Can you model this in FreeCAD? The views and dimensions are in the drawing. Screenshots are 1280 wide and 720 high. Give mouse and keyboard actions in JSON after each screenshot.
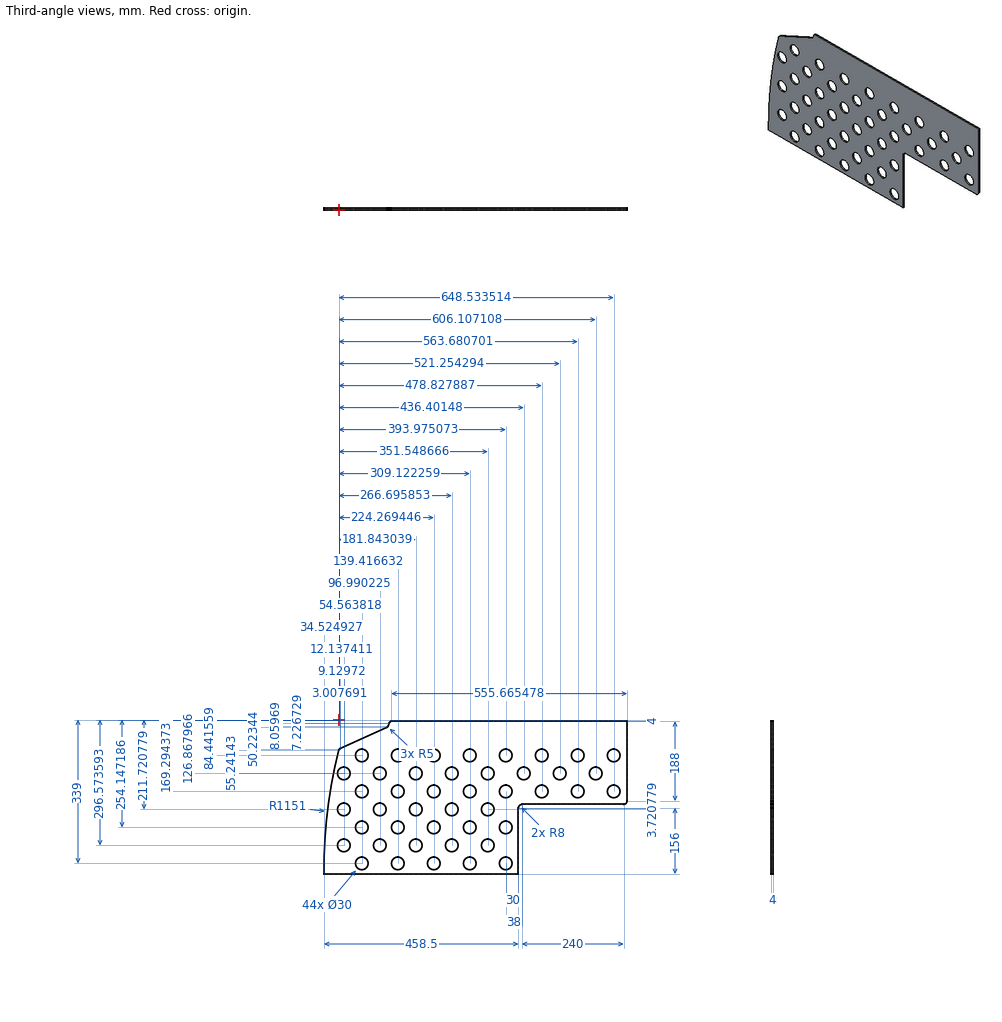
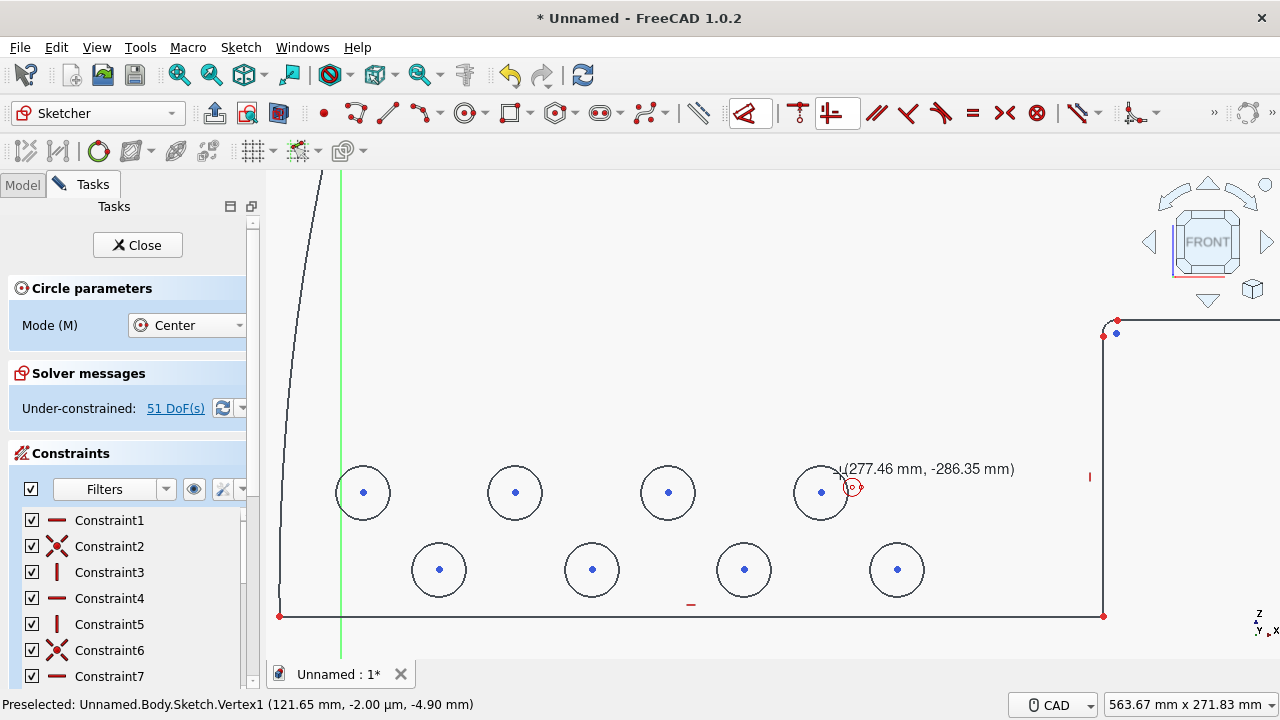
{"action": "left_click", "coordinate": [439, 416]}
{"action": "left_click", "coordinate": [458, 397]}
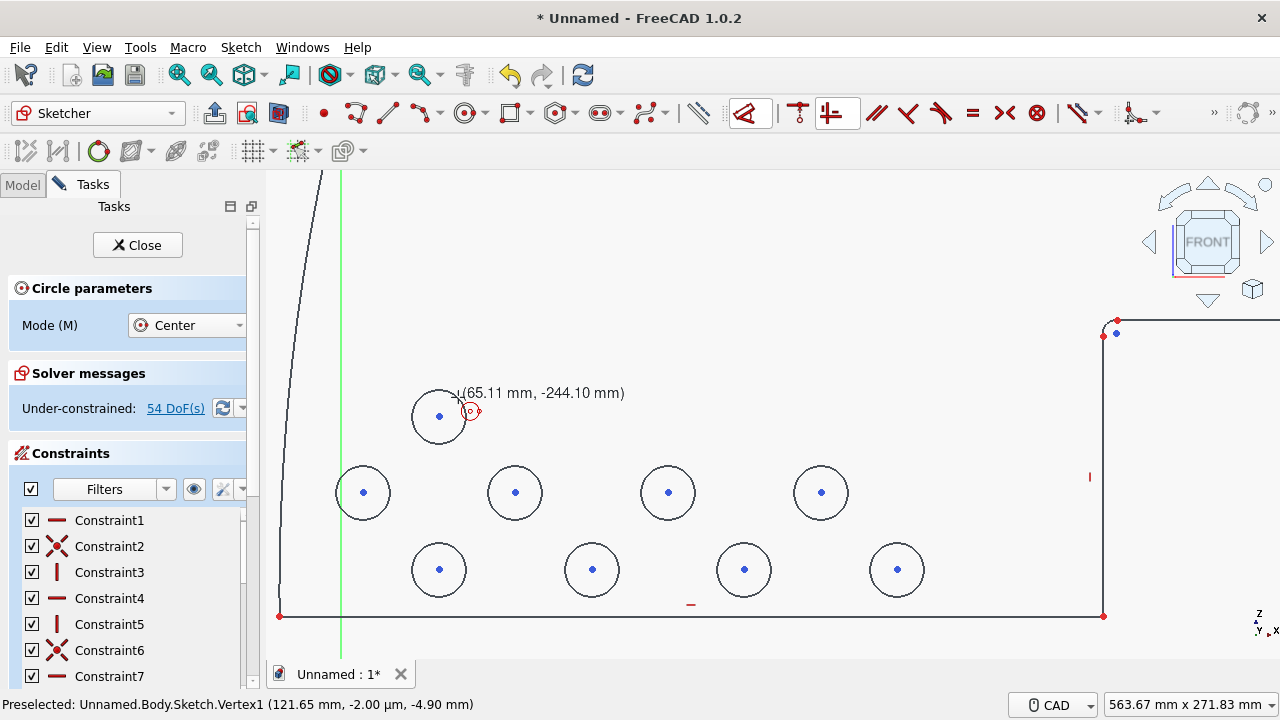
{"action": "left_click", "coordinate": [592, 416]}
{"action": "left_click", "coordinate": [611, 397]}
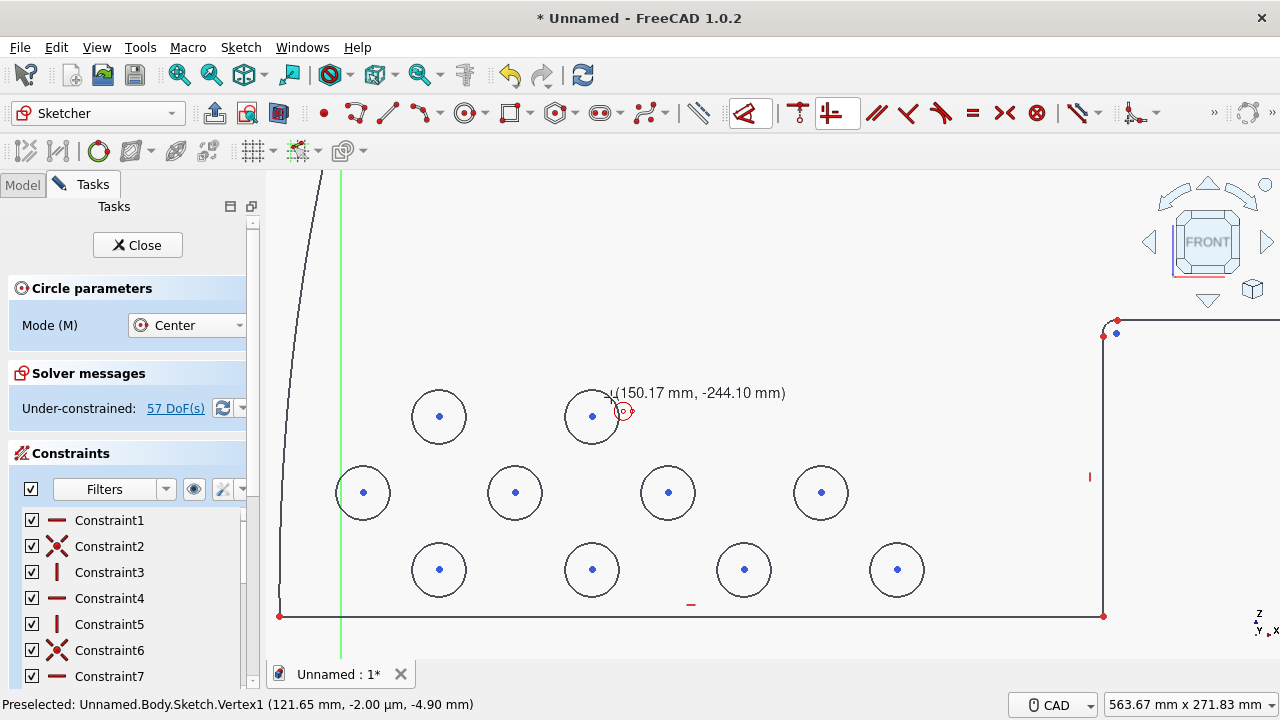
{"action": "left_click", "coordinate": [744, 416]}
{"action": "left_click", "coordinate": [763, 397]}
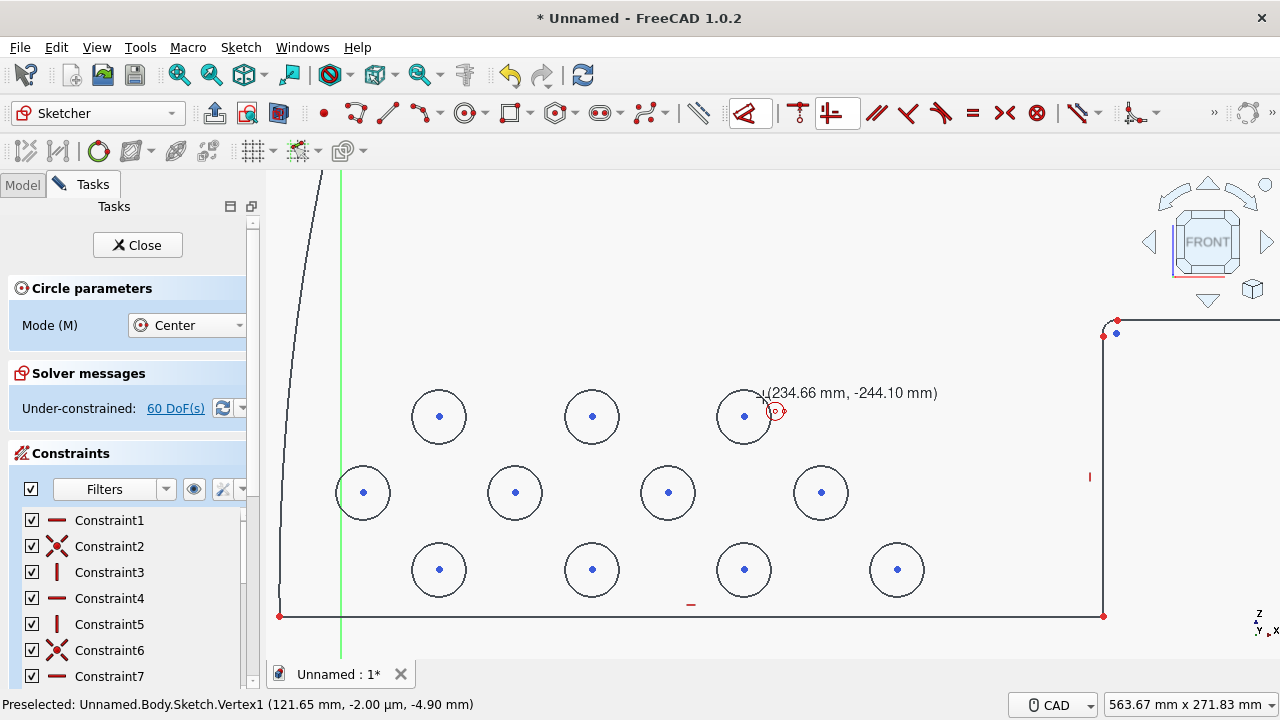
{"action": "left_click", "coordinate": [897, 416]}
{"action": "left_click", "coordinate": [916, 397]}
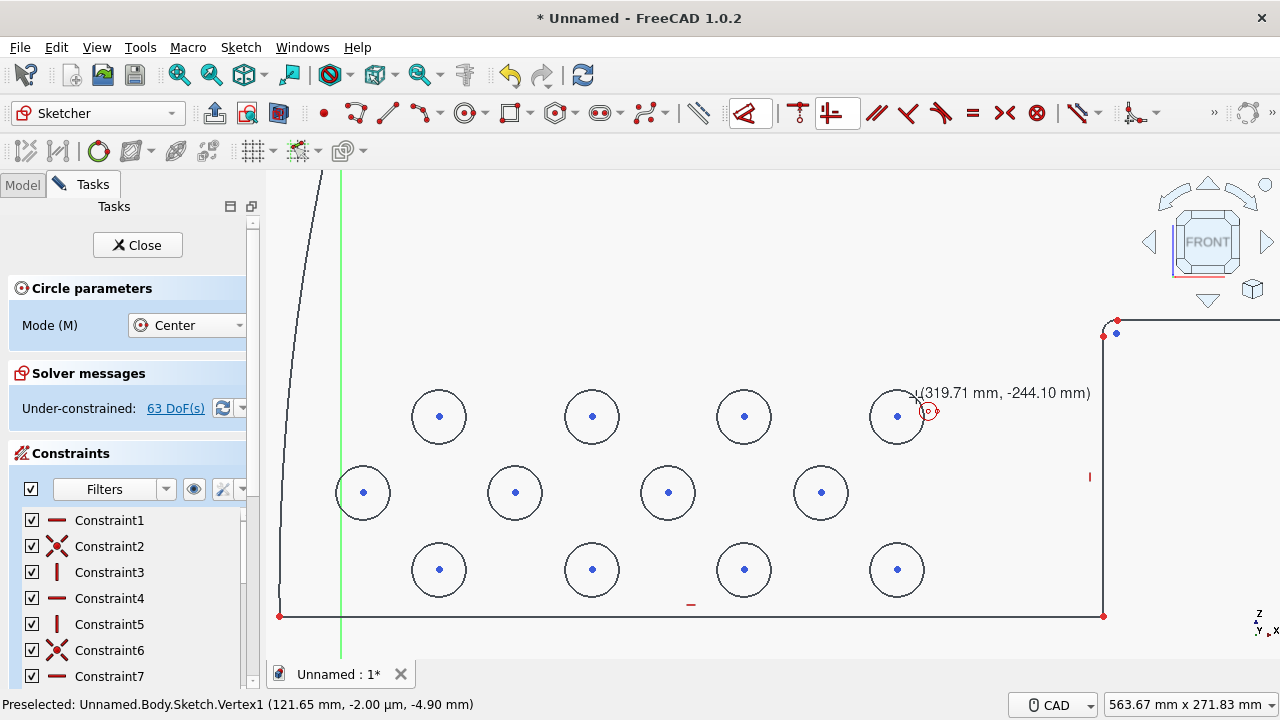
{"action": "left_click", "coordinate": [1050, 569]}
{"action": "left_click", "coordinate": [1069, 550]}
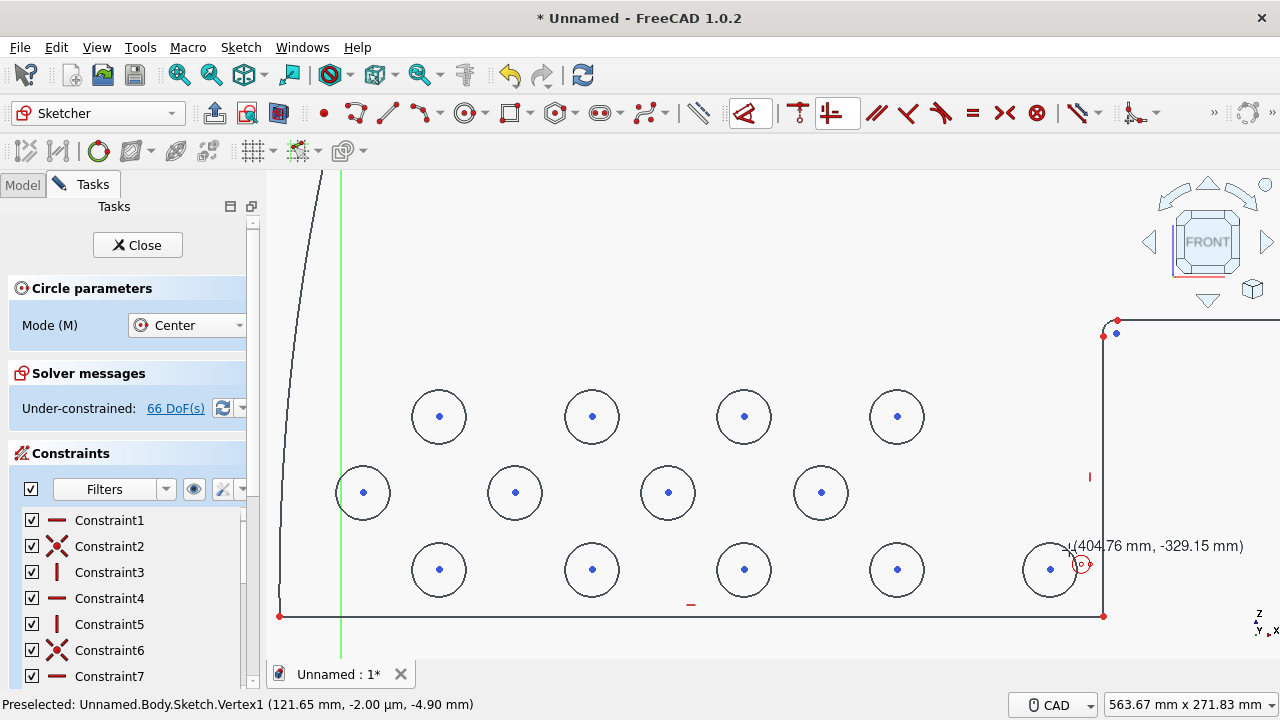
{"action": "left_click", "coordinate": [973, 492]}
{"action": "left_click", "coordinate": [992, 473]}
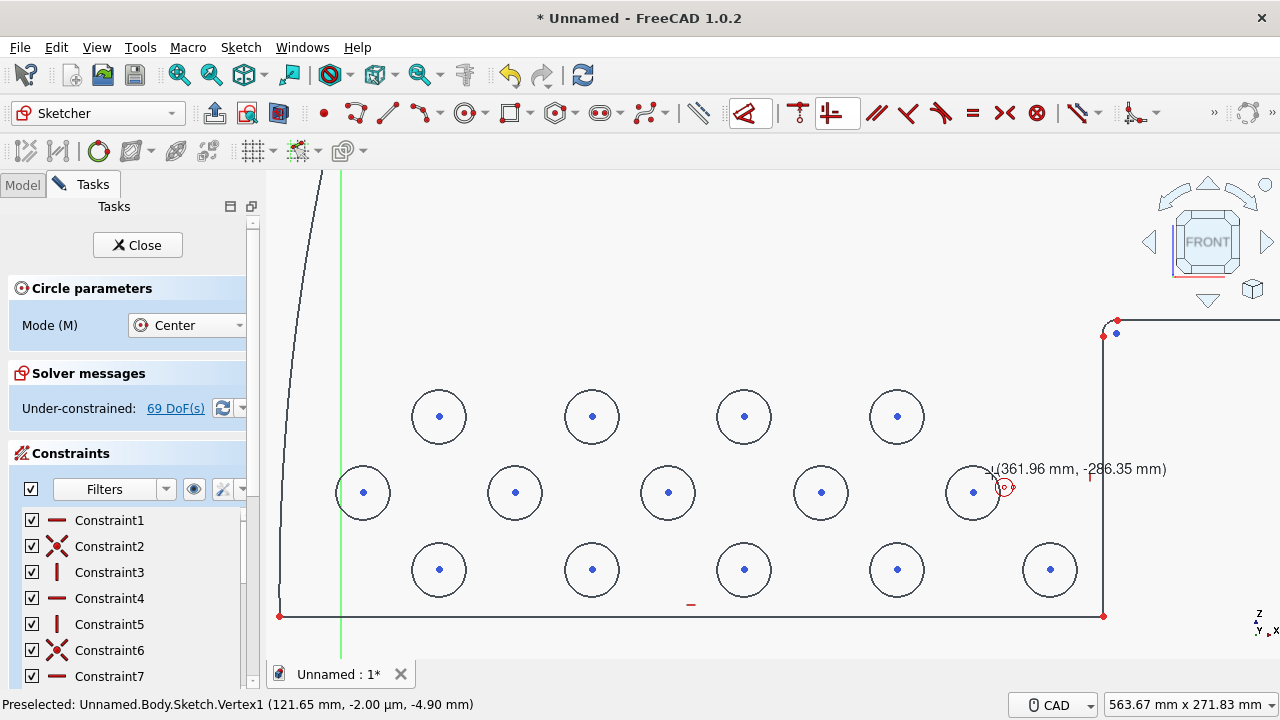
{"action": "left_click", "coordinate": [1050, 416]}
{"action": "left_click", "coordinate": [1069, 397]}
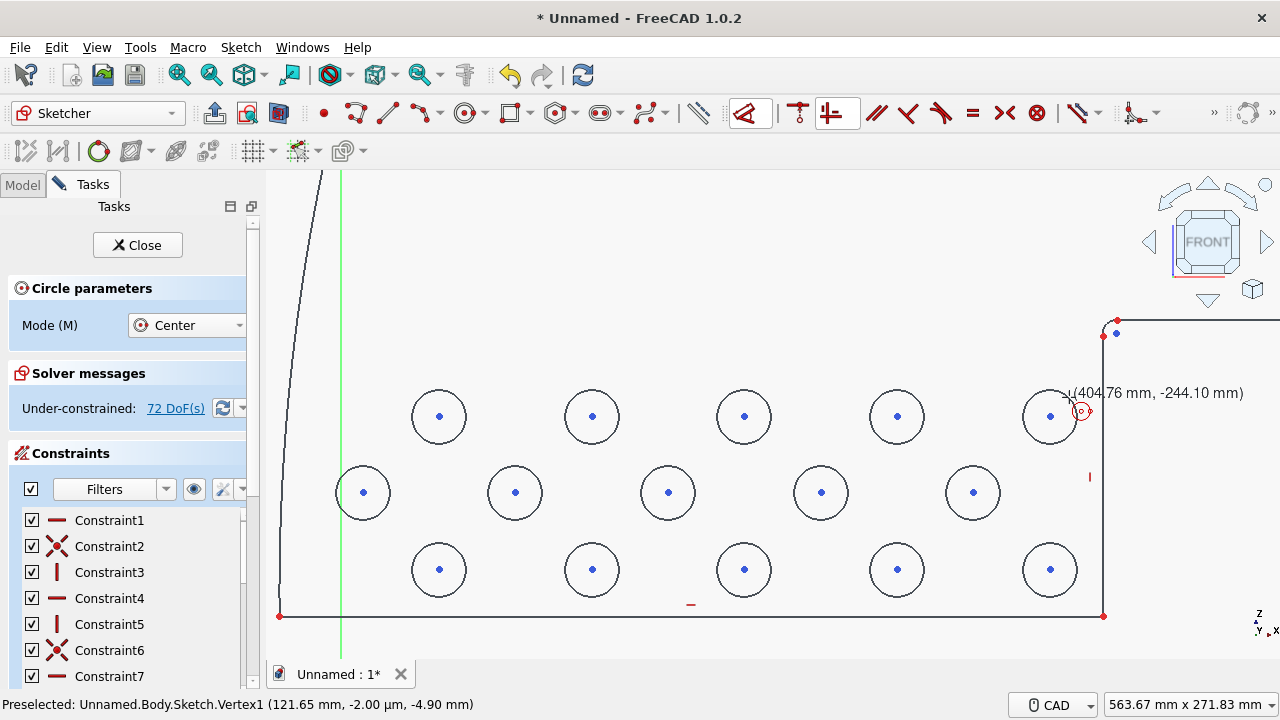
{"action": "left_click", "coordinate": [363, 340]}
{"action": "left_click", "coordinate": [382, 321]}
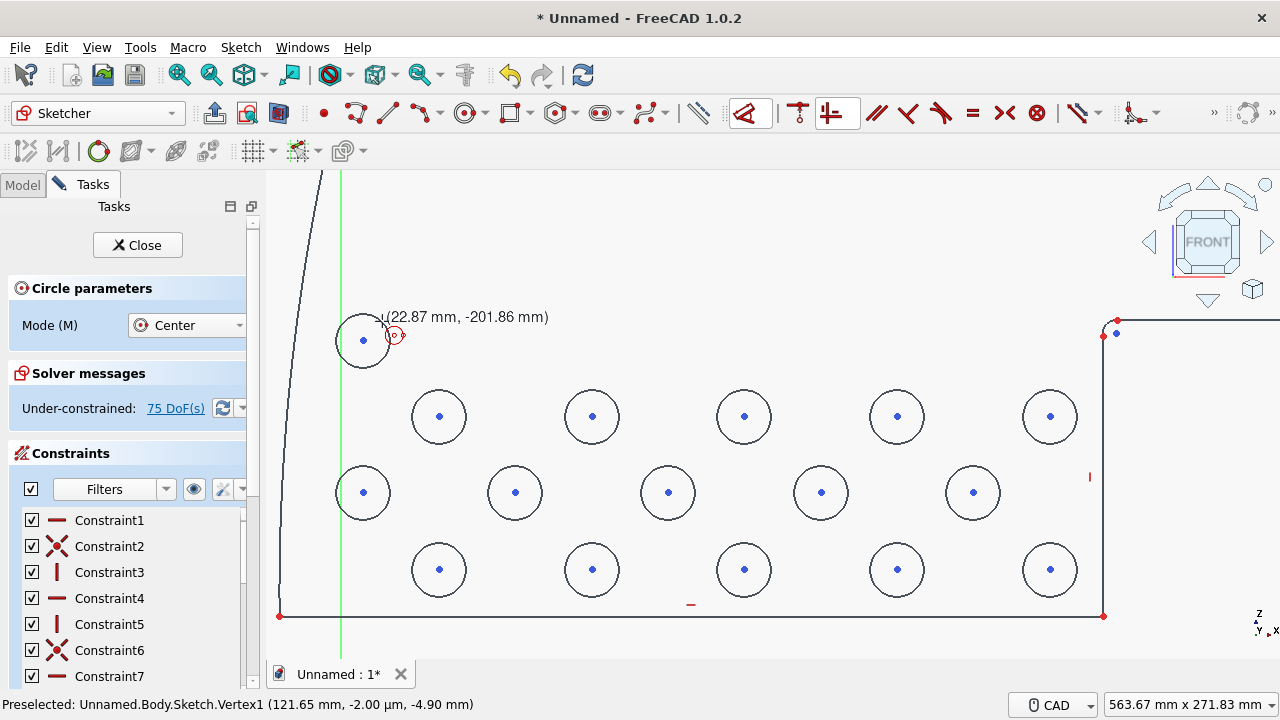
{"action": "left_click", "coordinate": [515, 340]}
{"action": "left_click", "coordinate": [534, 321]}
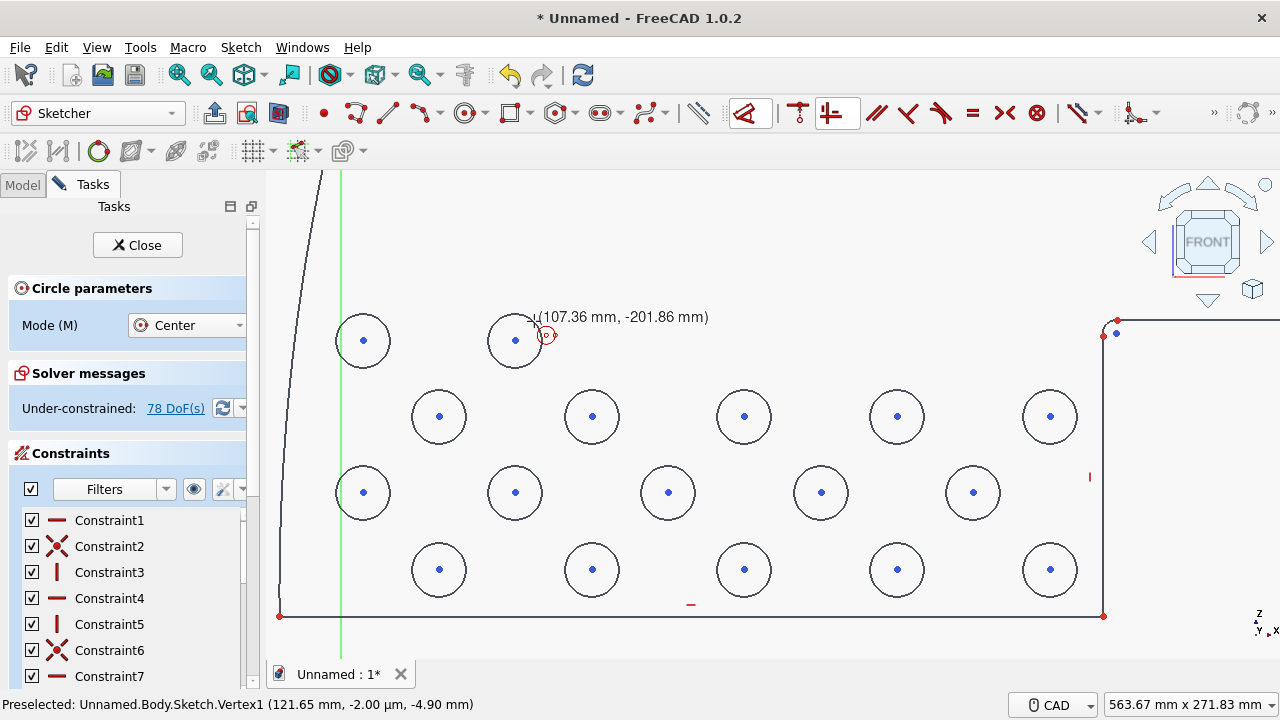
{"action": "left_click", "coordinate": [439, 263]}
{"action": "left_click", "coordinate": [458, 244]}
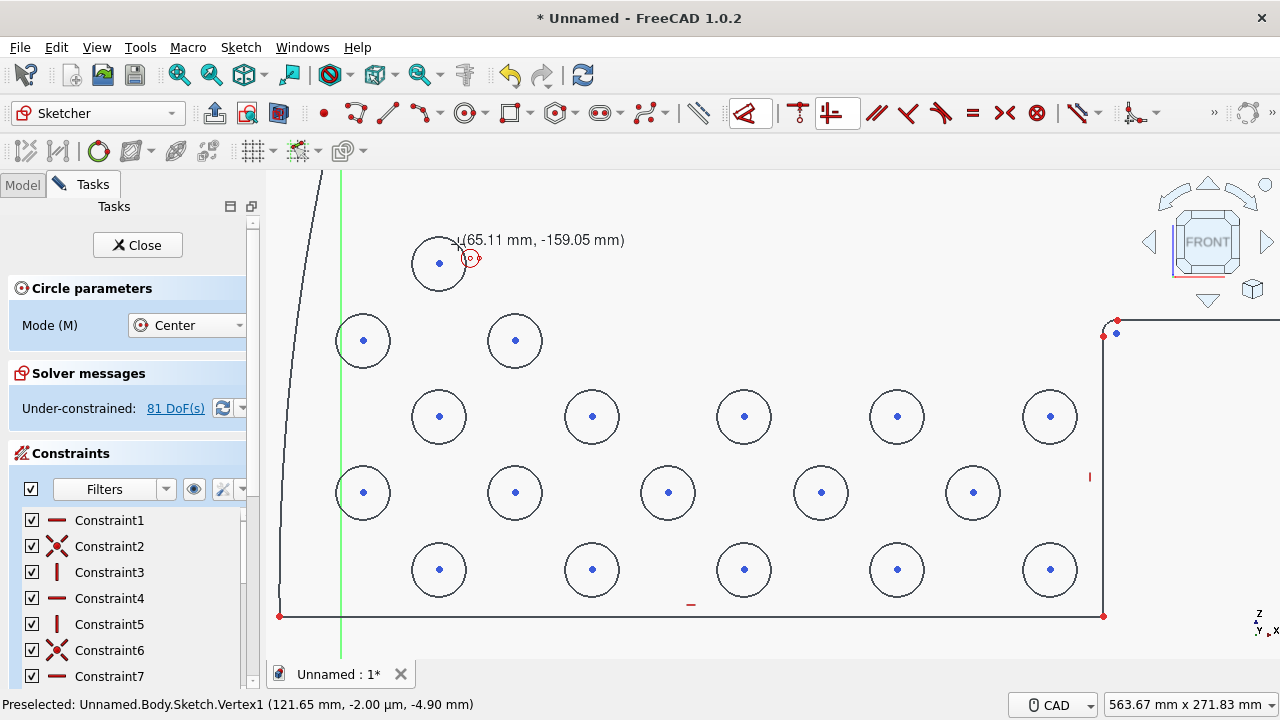
{"action": "left_click", "coordinate": [592, 263]}
{"action": "left_click", "coordinate": [611, 244]}